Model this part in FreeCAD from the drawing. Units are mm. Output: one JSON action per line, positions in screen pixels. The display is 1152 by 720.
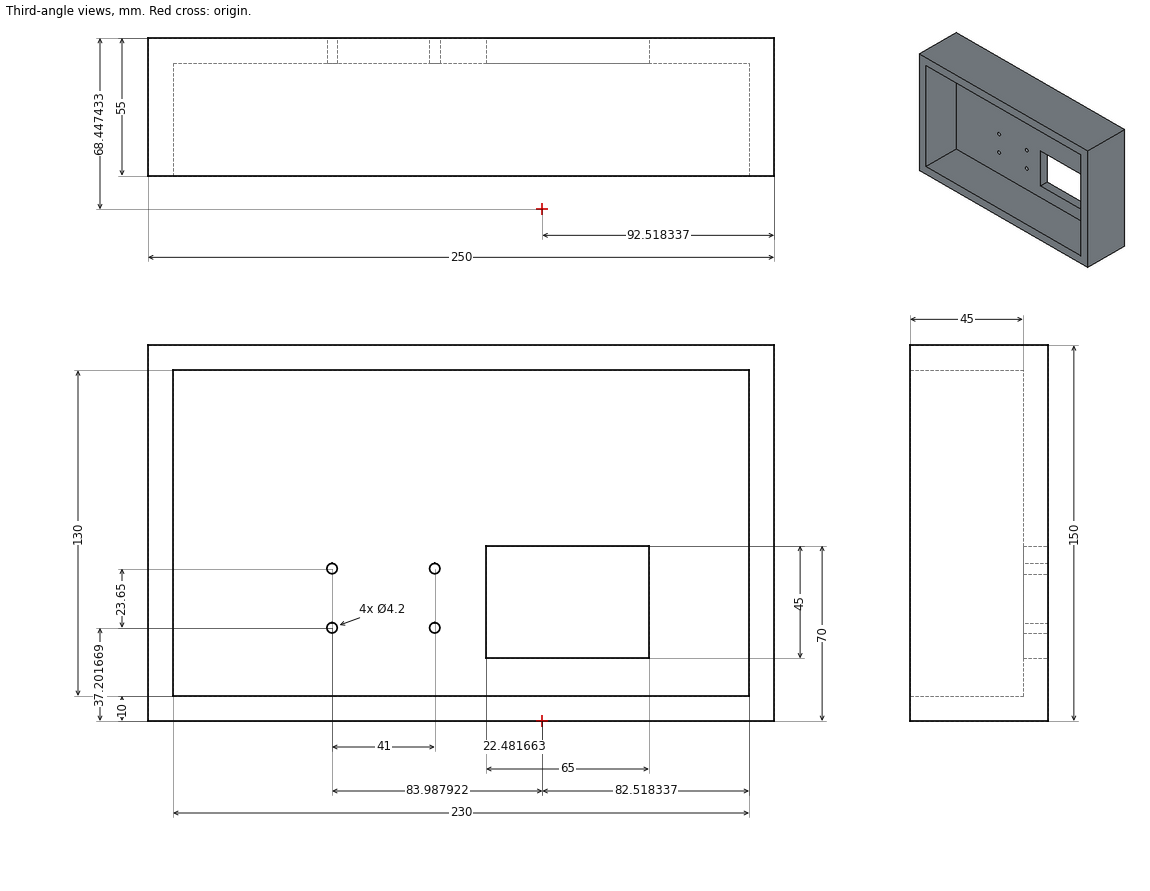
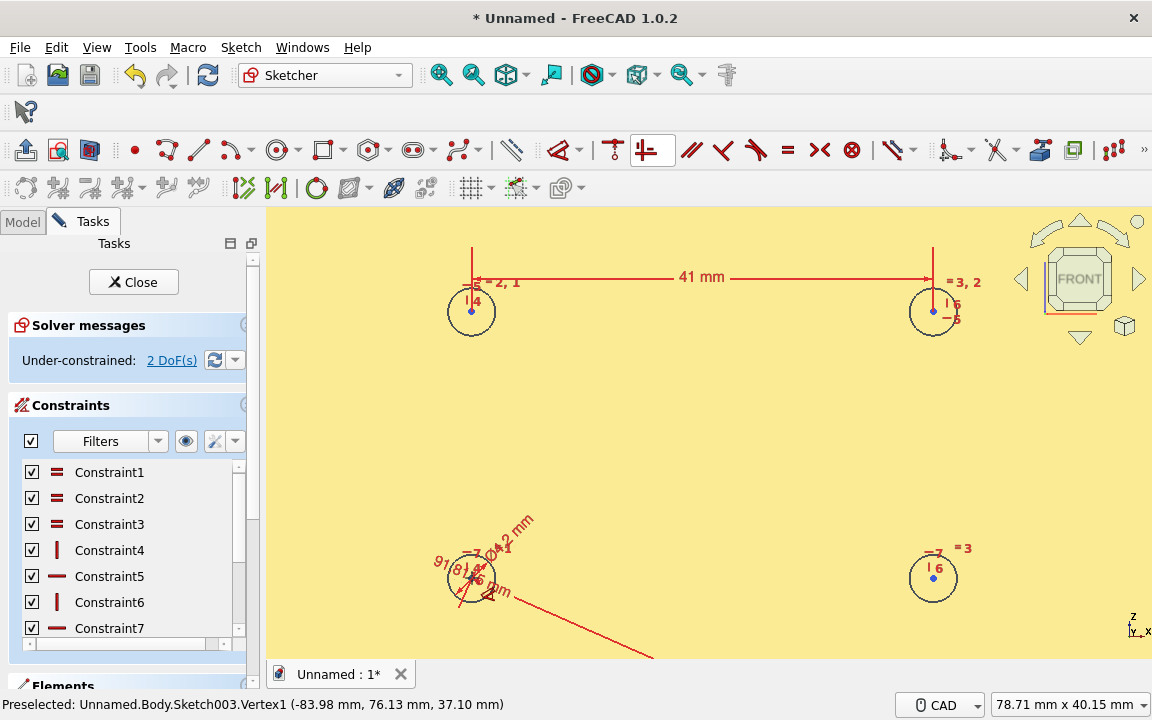
{"action": "left_click", "coordinate": [472, 312]}
{"action": "left_click", "coordinate": [438, 445]}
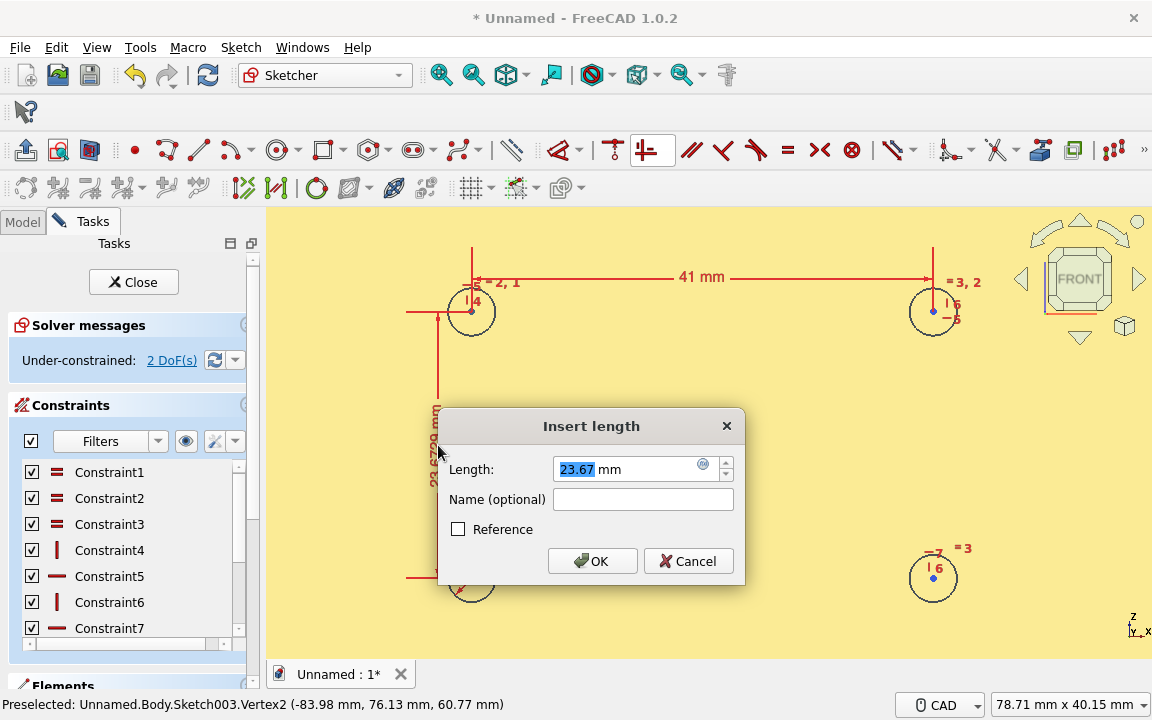
{"action": "type", "text": "23.65"}
{"action": "key", "text": "Return"}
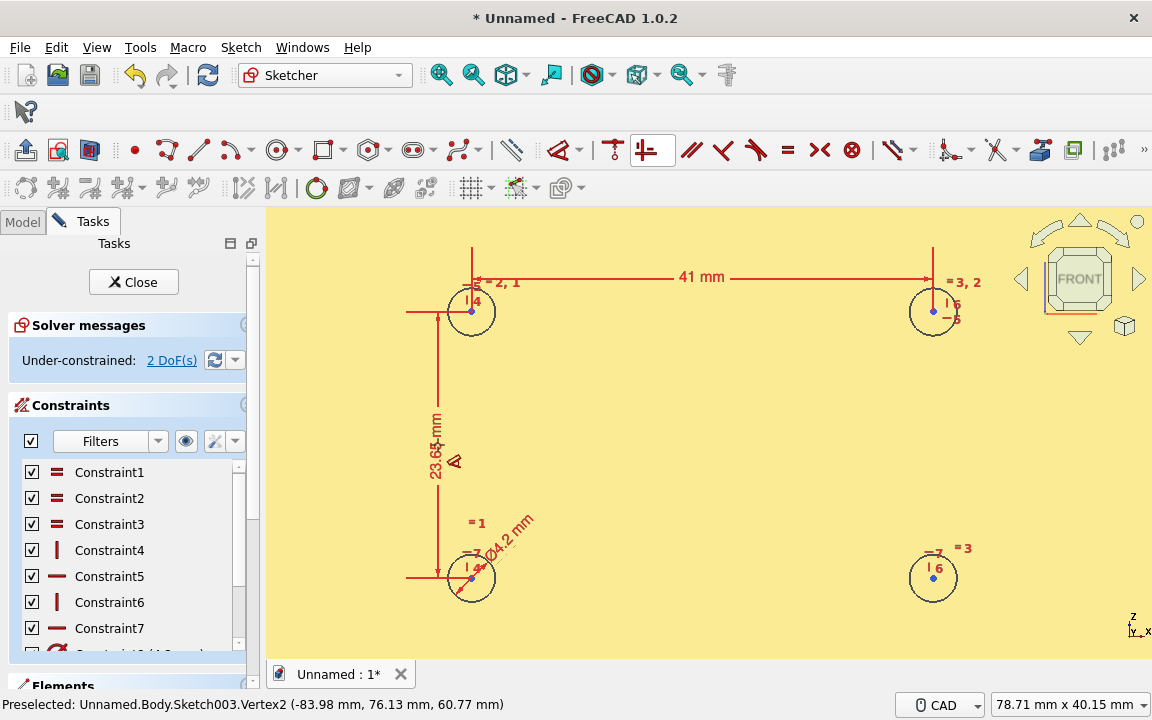
{"action": "left_click", "coordinate": [472, 578]}
{"action": "left_click", "coordinate": [729, 544]}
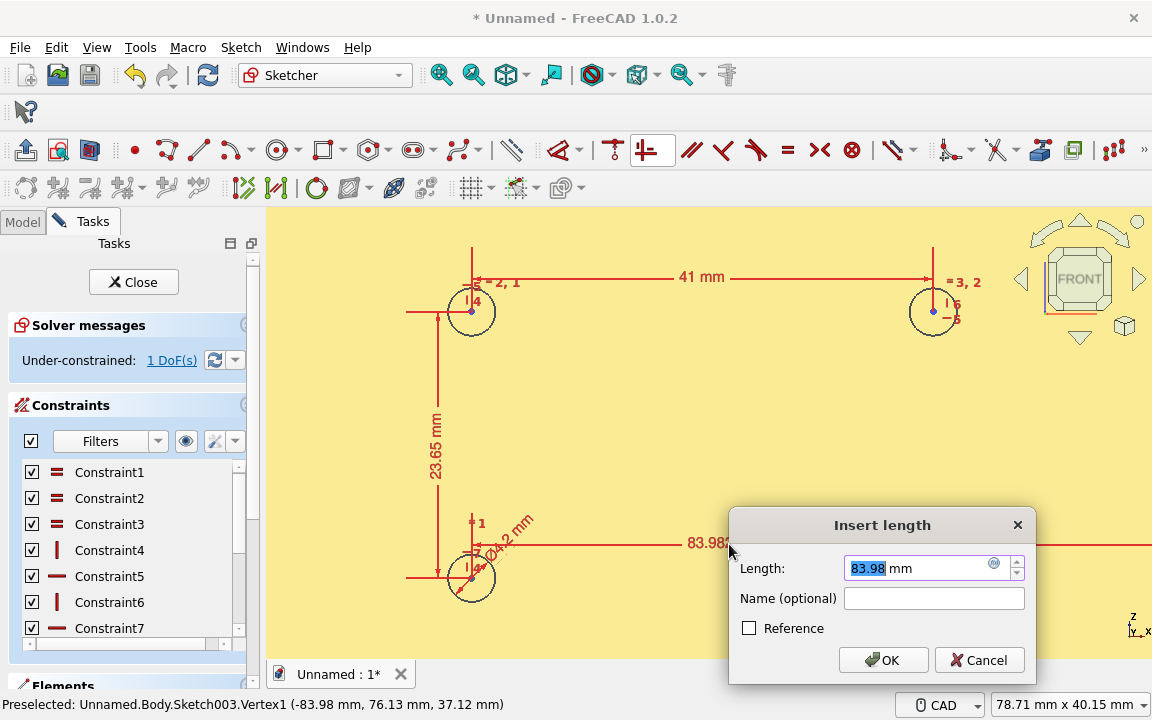
{"action": "type", "text": "83.987922"}
{"action": "key", "text": "Return"}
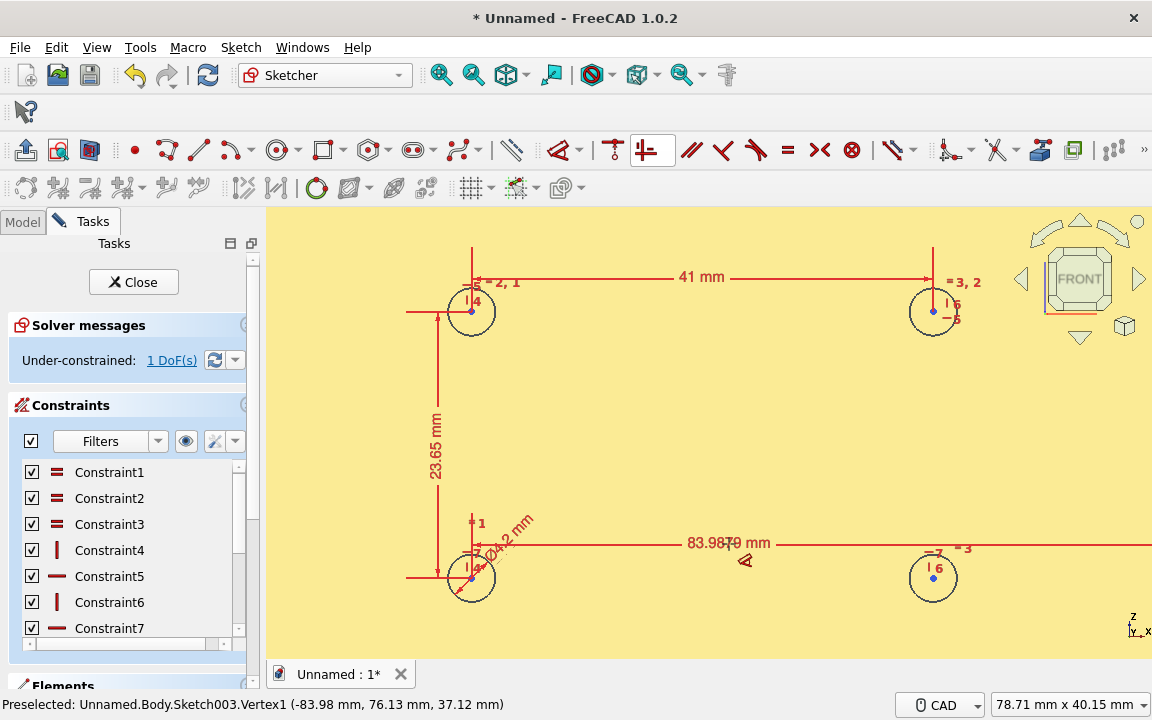
{"action": "left_click", "coordinate": [472, 578]}
{"action": "left_click", "coordinate": [438, 605]}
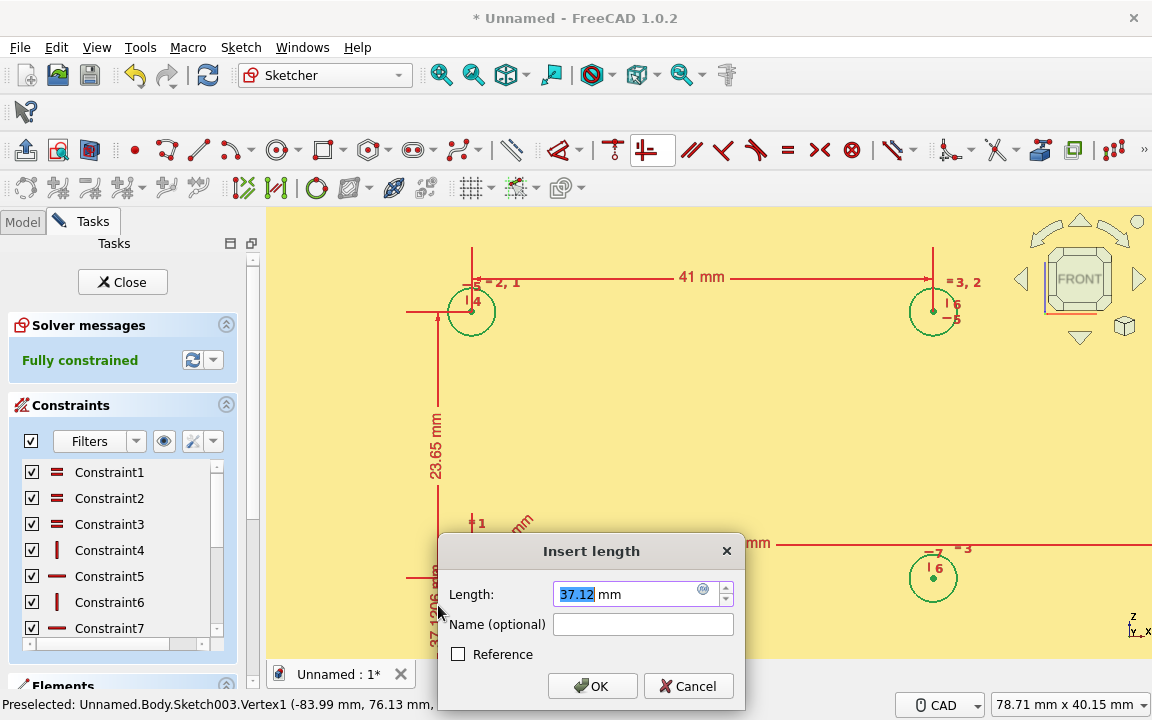
{"action": "type", "text": "37.201669"}
{"action": "key", "text": "Return"}
{"action": "key", "text": "Escape"}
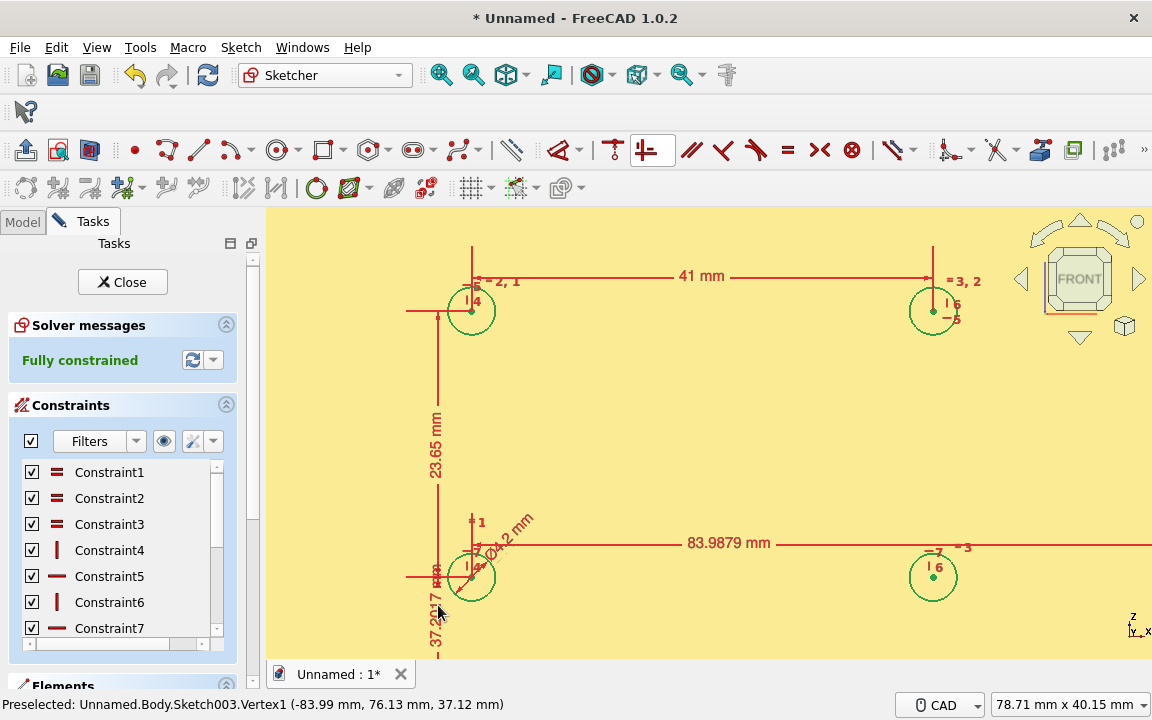
{"action": "left_click", "coordinate": [123, 282]}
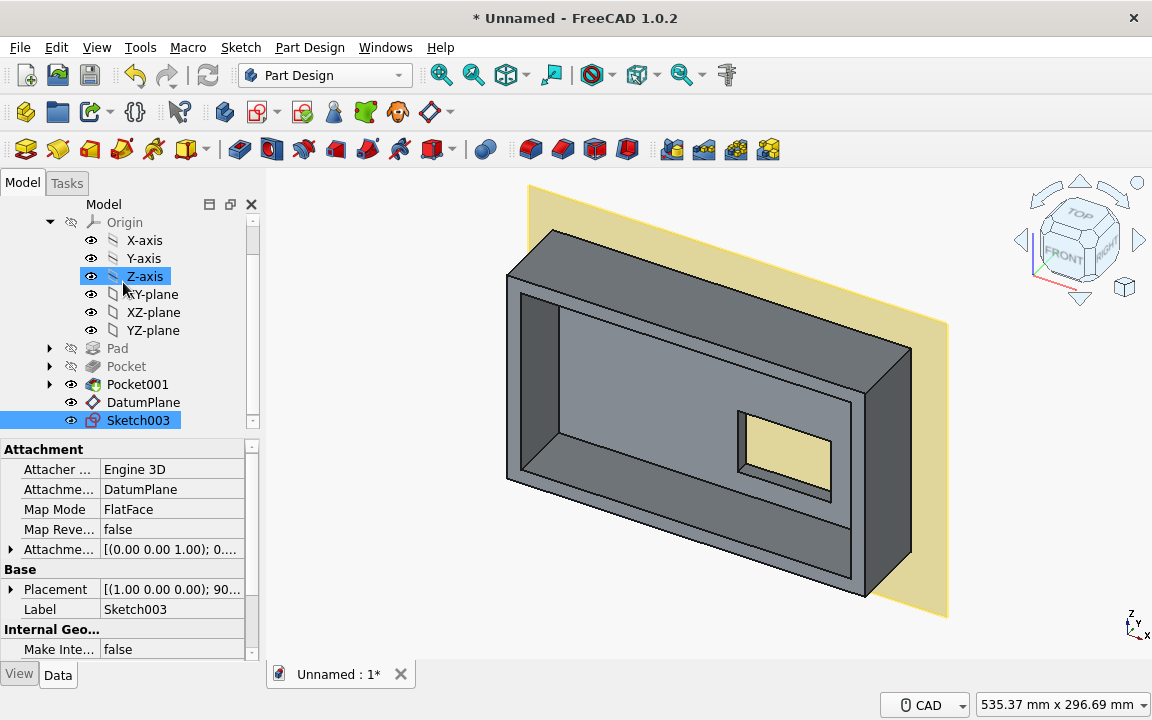
{"action": "left_click", "coordinate": [240, 150]}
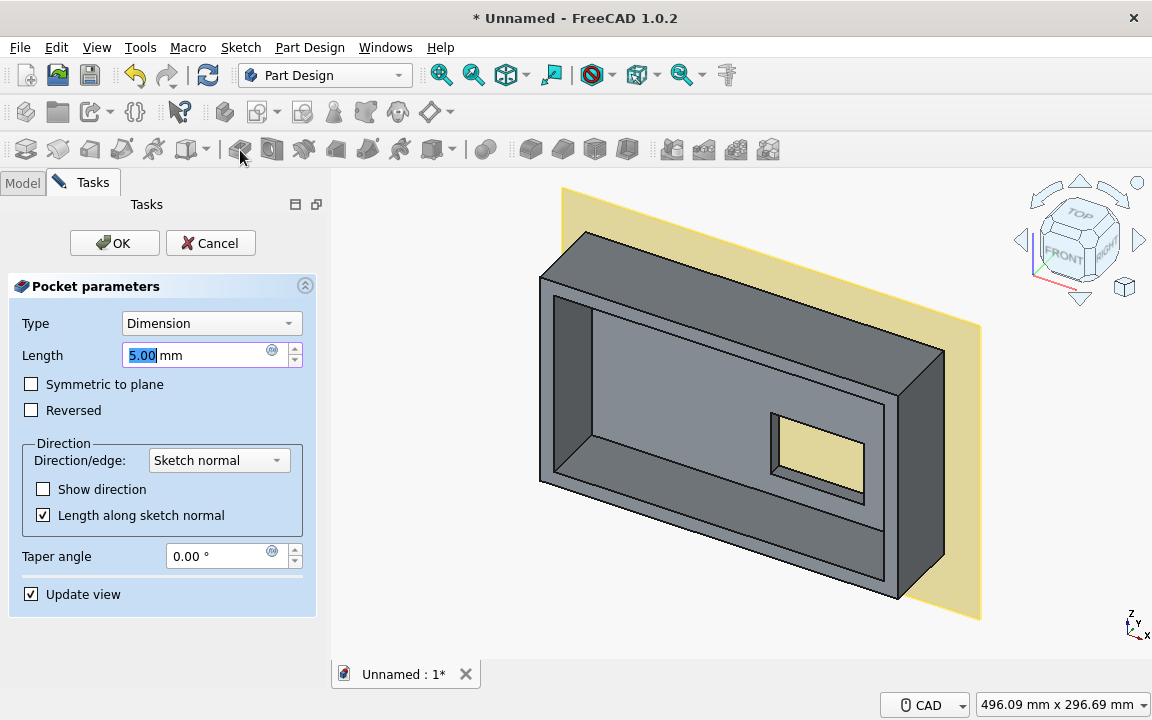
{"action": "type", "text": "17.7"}
{"action": "key", "text": "Tab"}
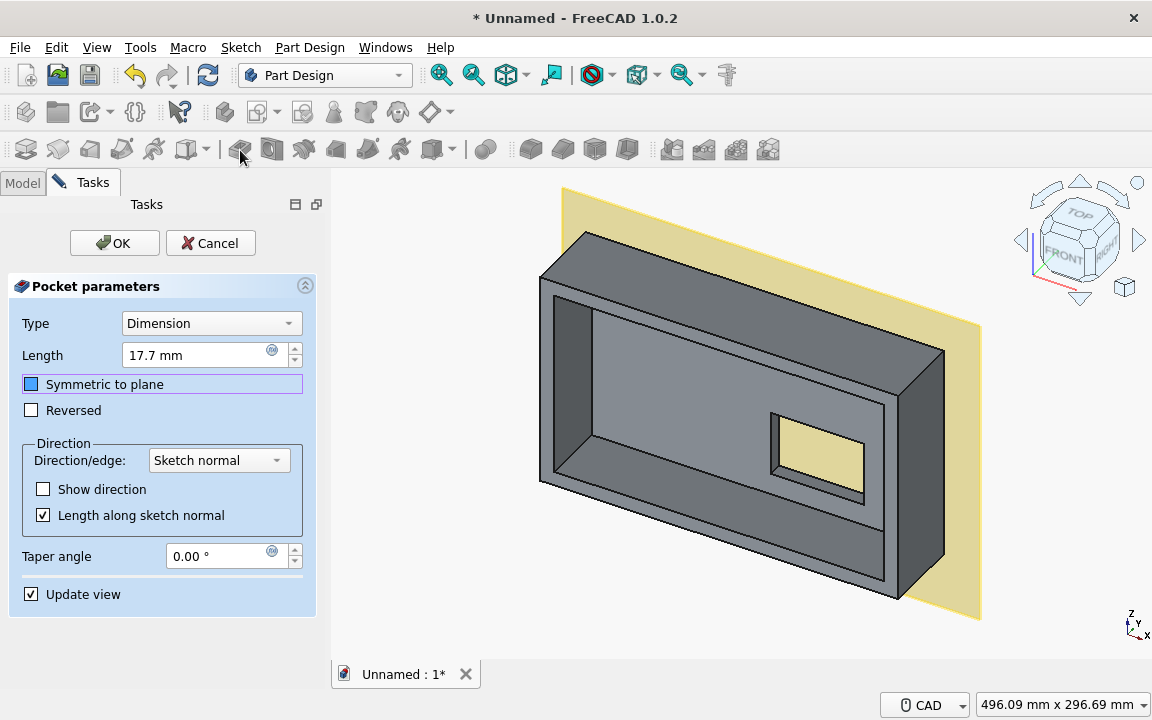
{"action": "left_click", "coordinate": [30, 410]}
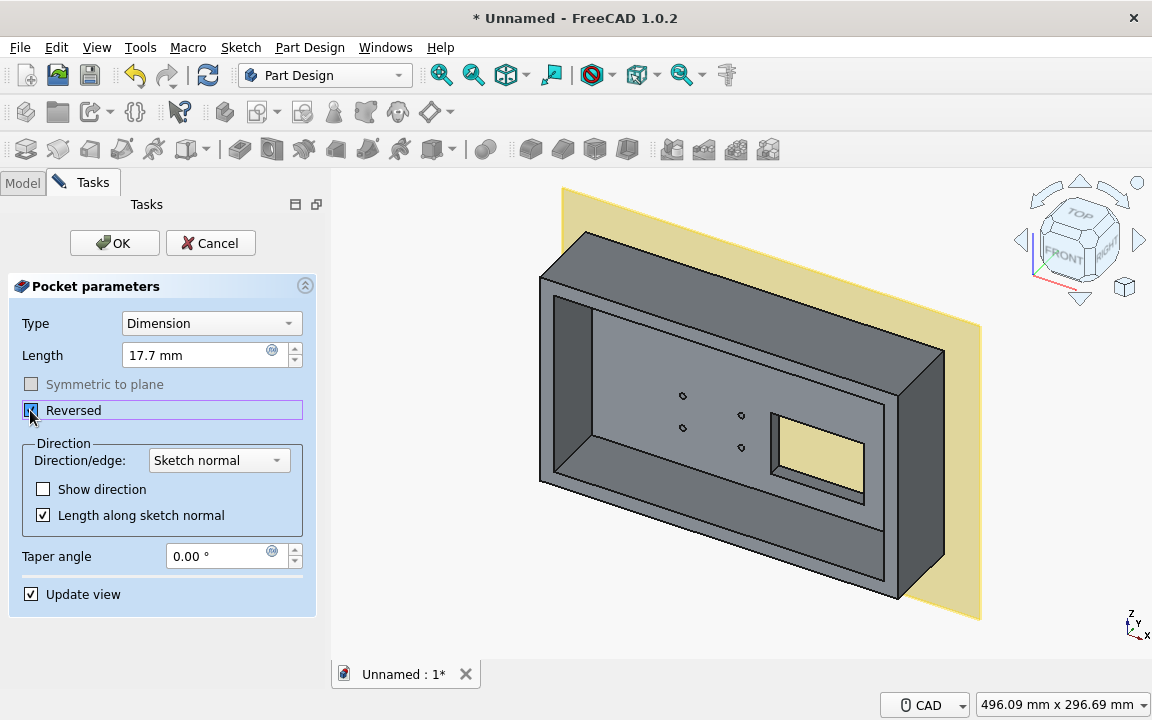
{"action": "left_click", "coordinate": [115, 243]}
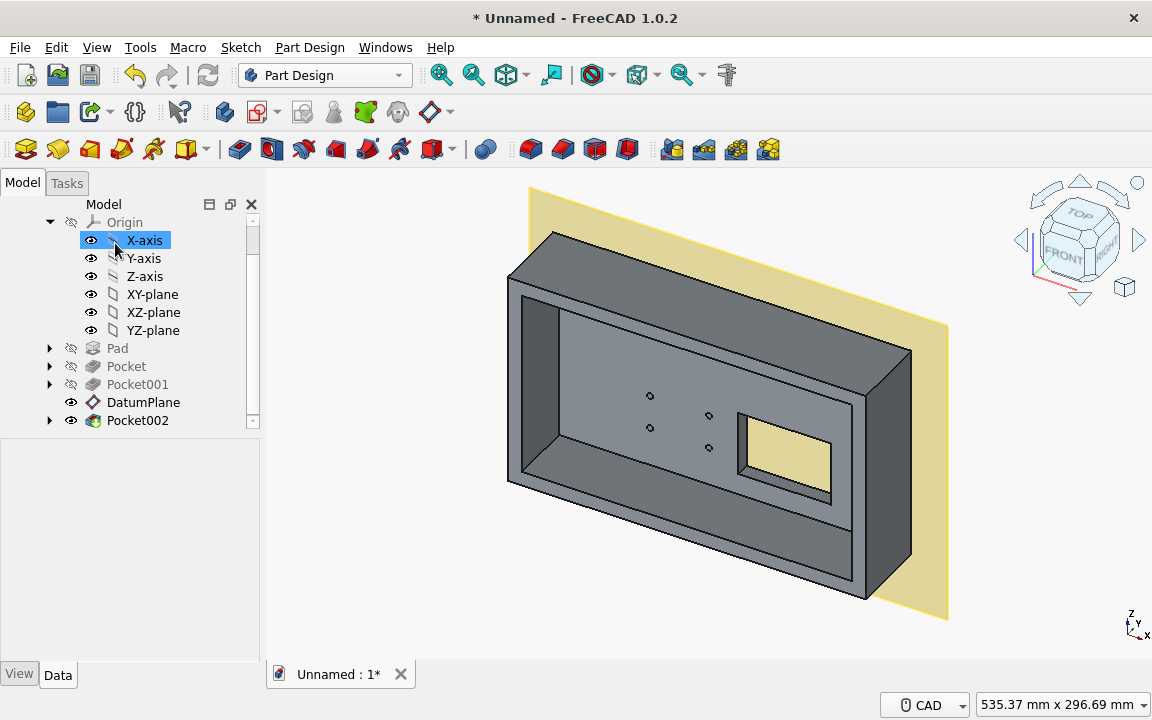
{"action": "left_click", "coordinate": [116, 402]}
{"action": "key", "text": "space"}